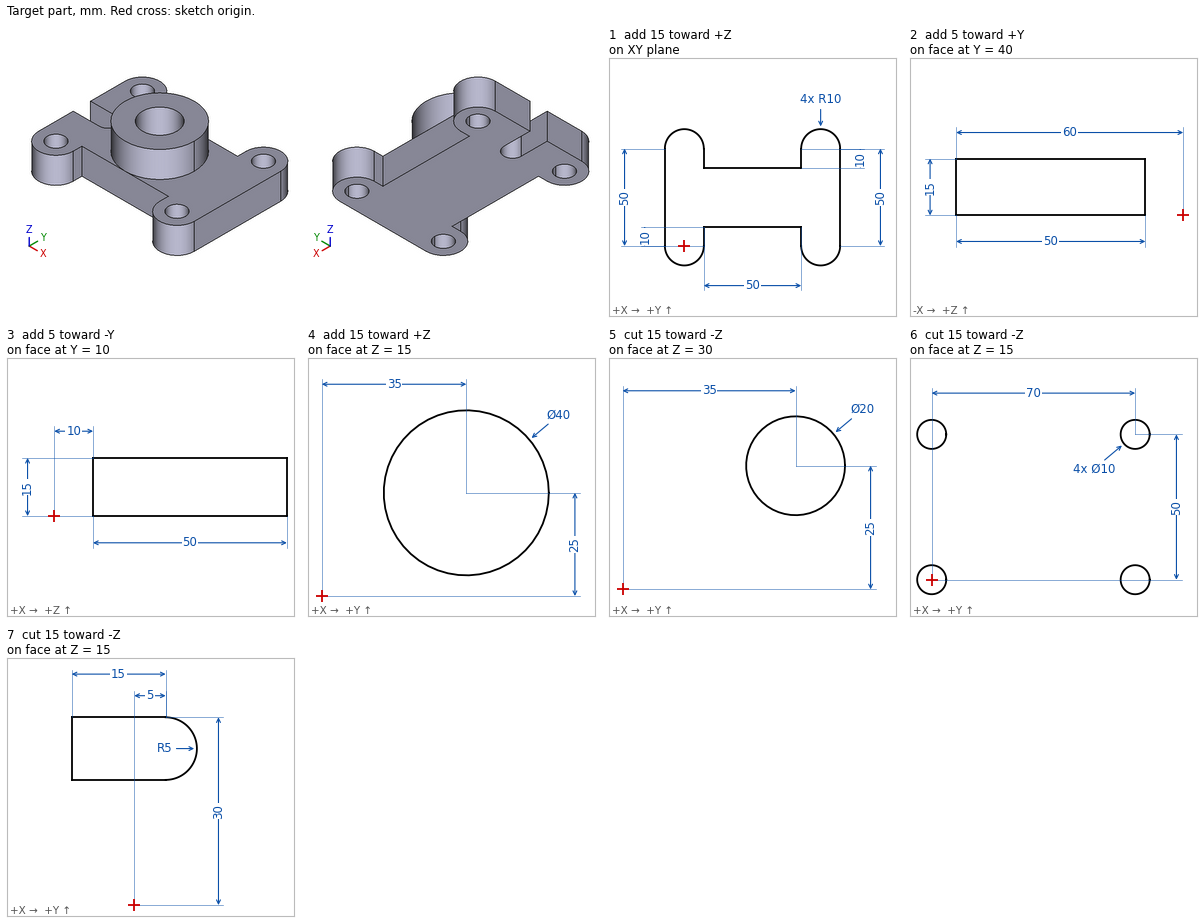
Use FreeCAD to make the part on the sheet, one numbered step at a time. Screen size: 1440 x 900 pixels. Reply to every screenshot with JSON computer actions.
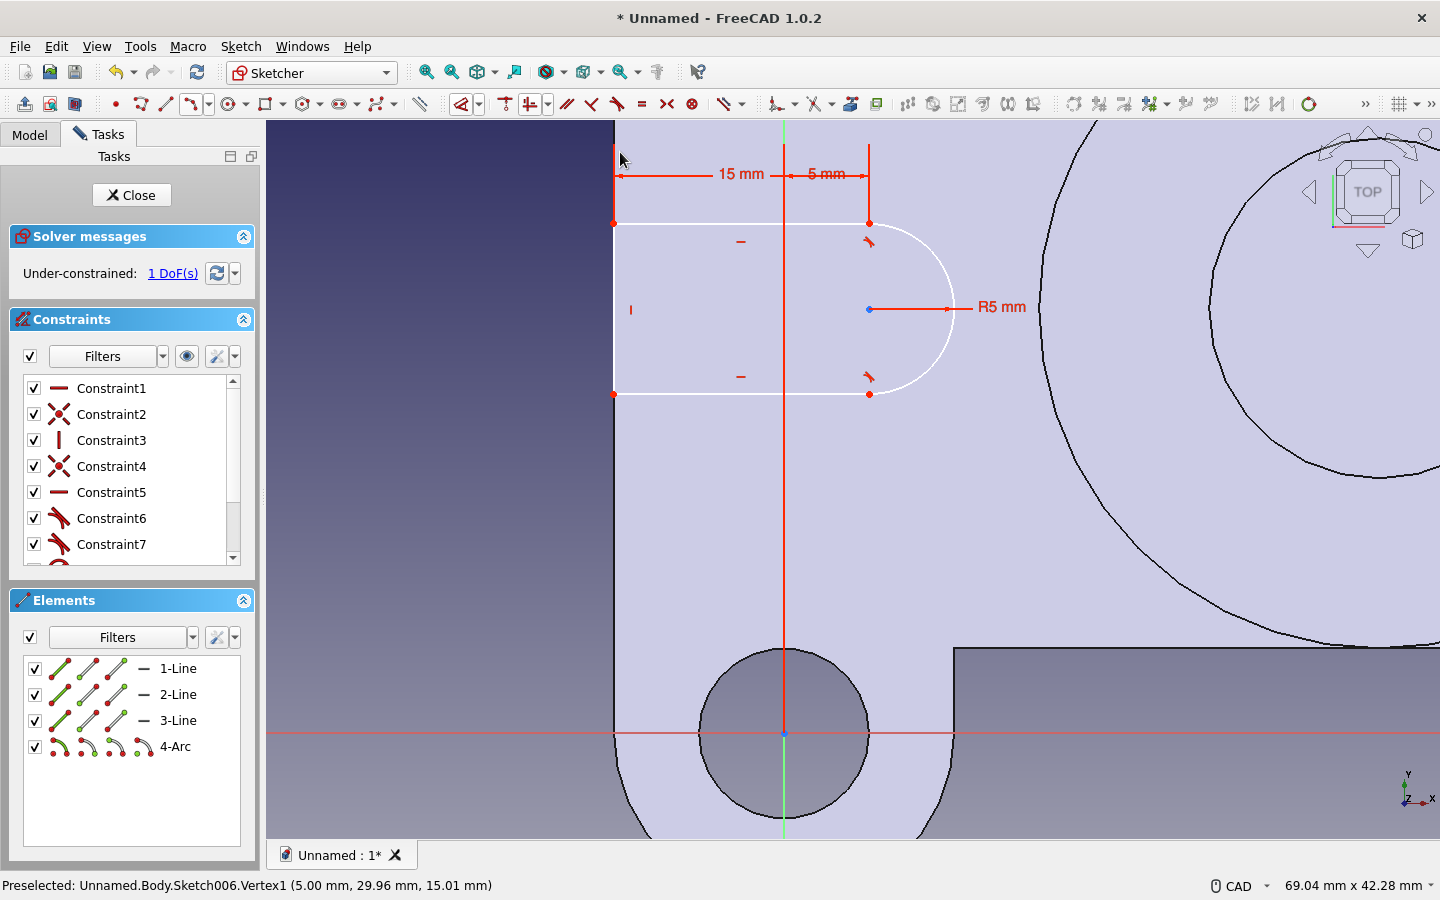
{"action": "left_click", "coordinate": [869, 224]}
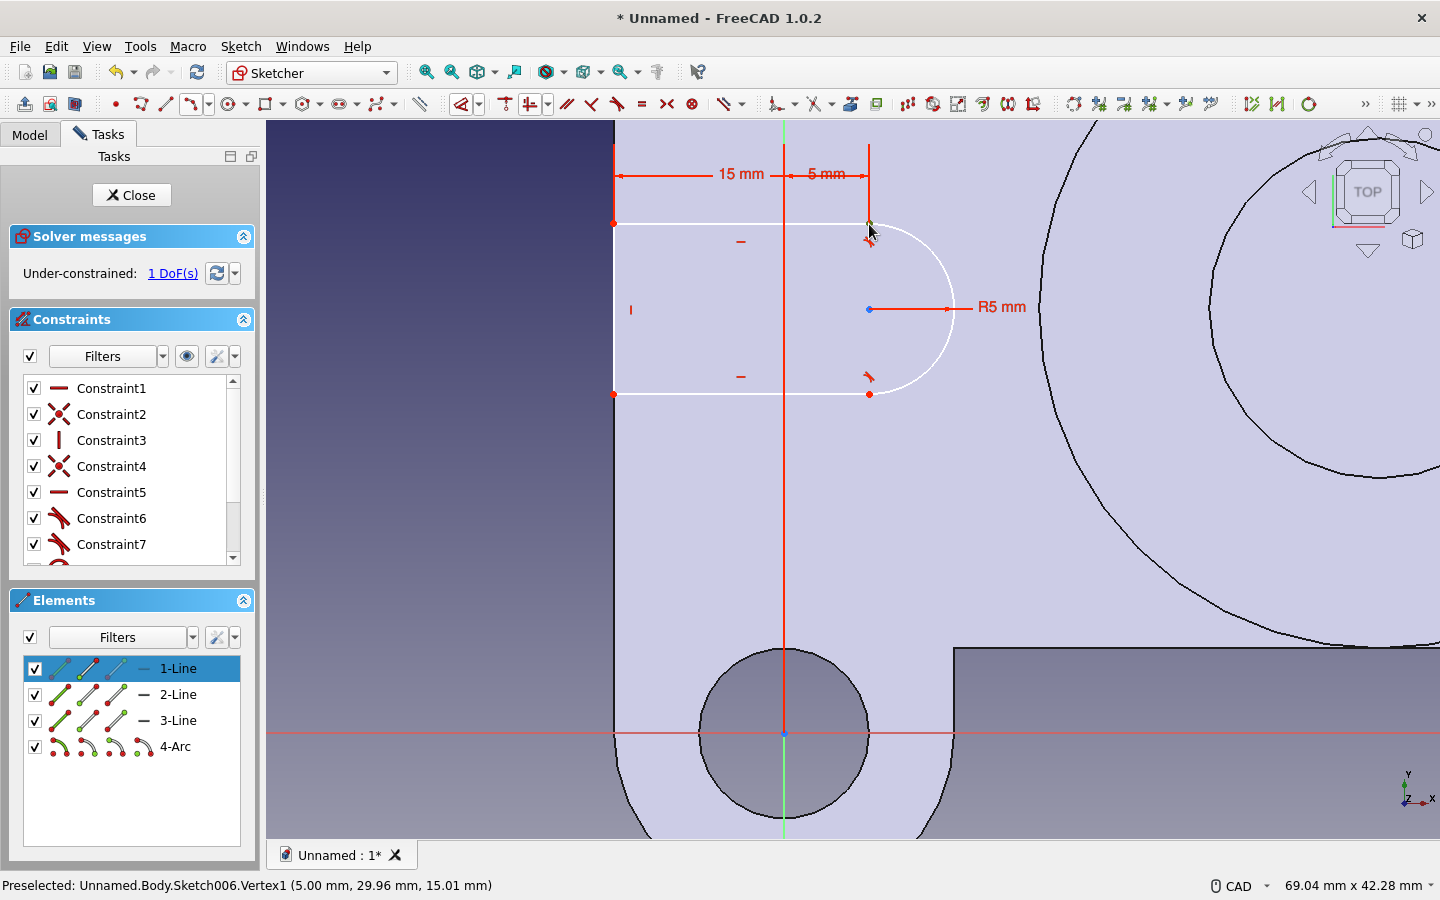
{"action": "key", "text": "i"}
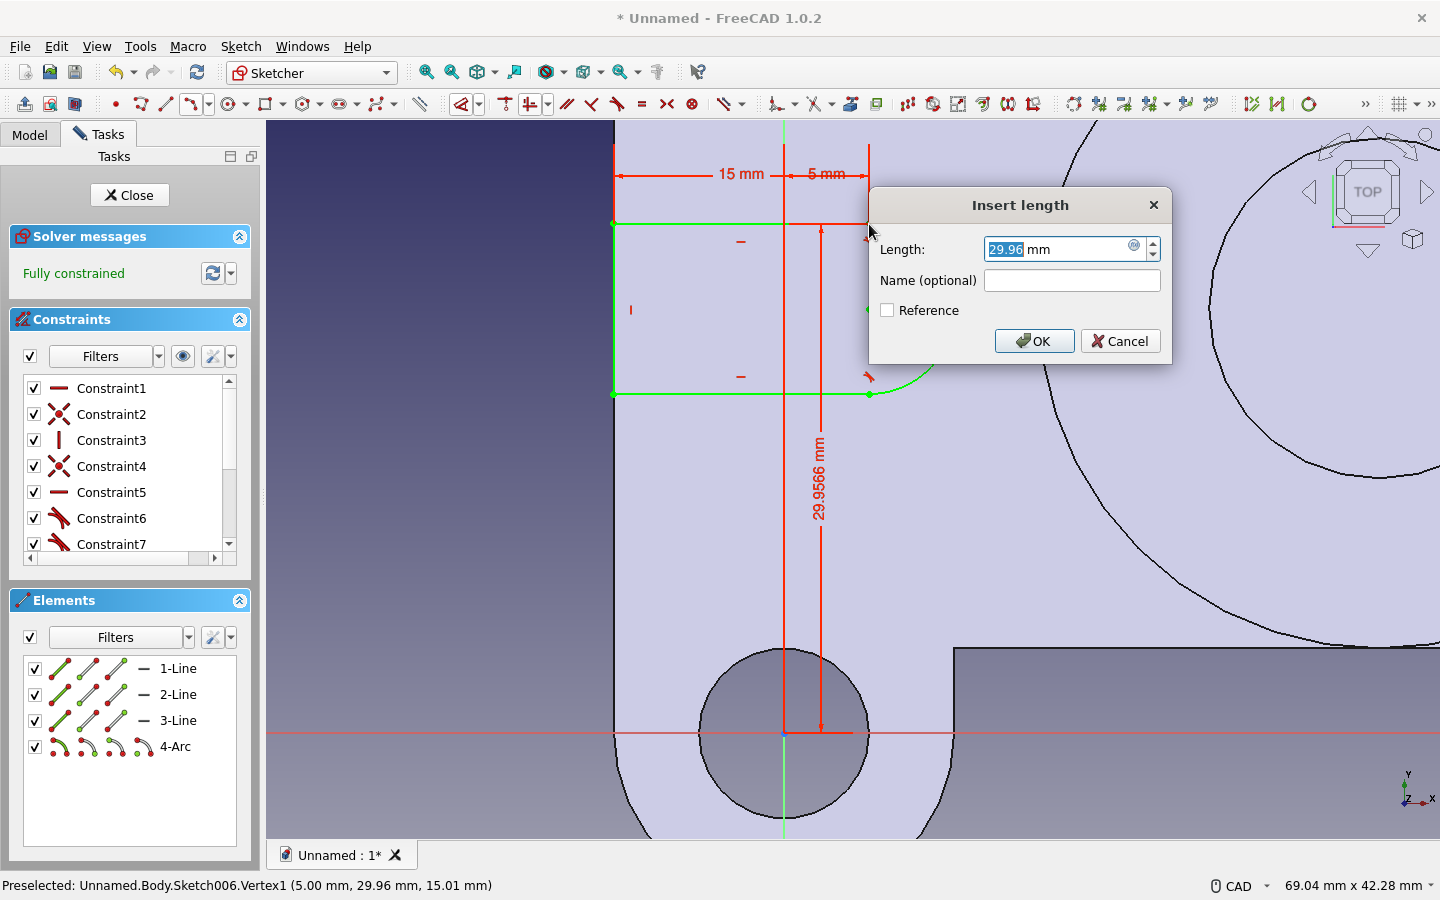
{"action": "type", "text": "30"}
{"action": "key", "text": "Return"}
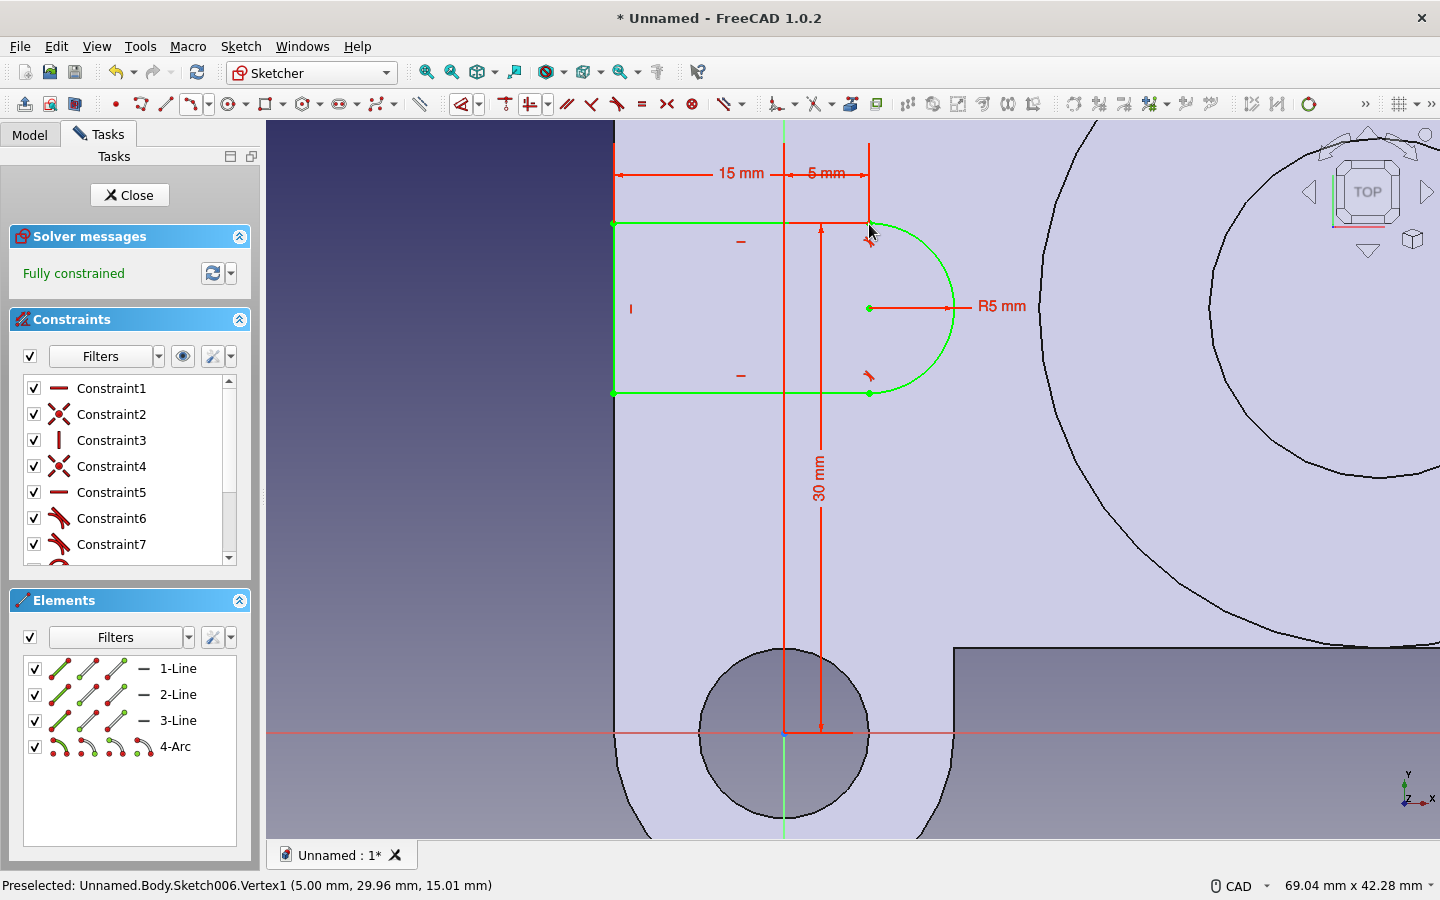
{"action": "left_click", "coordinate": [130, 195]}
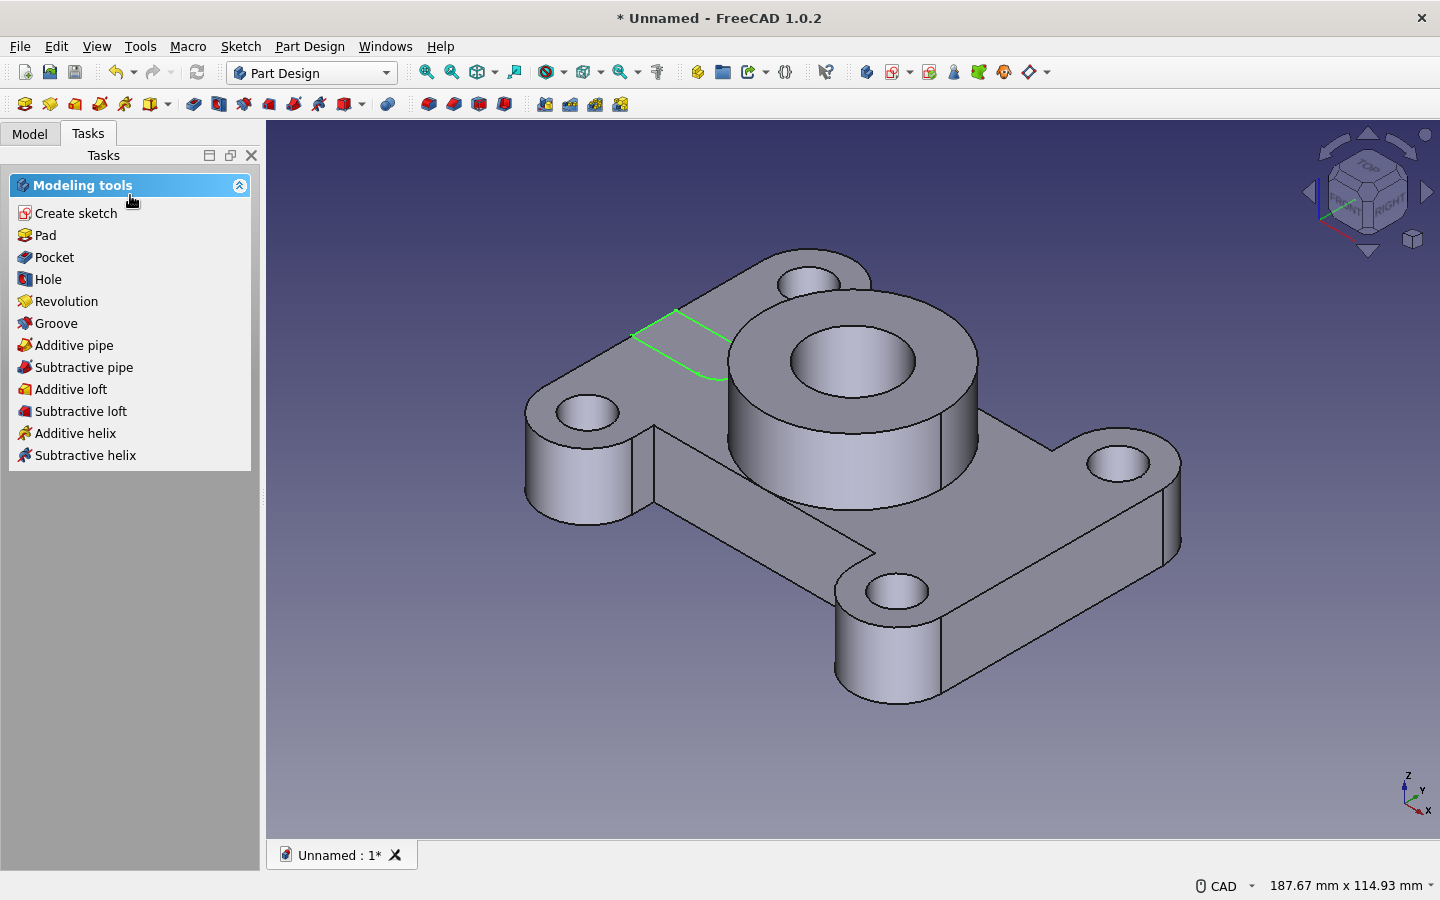
{"action": "left_click", "coordinate": [194, 104]}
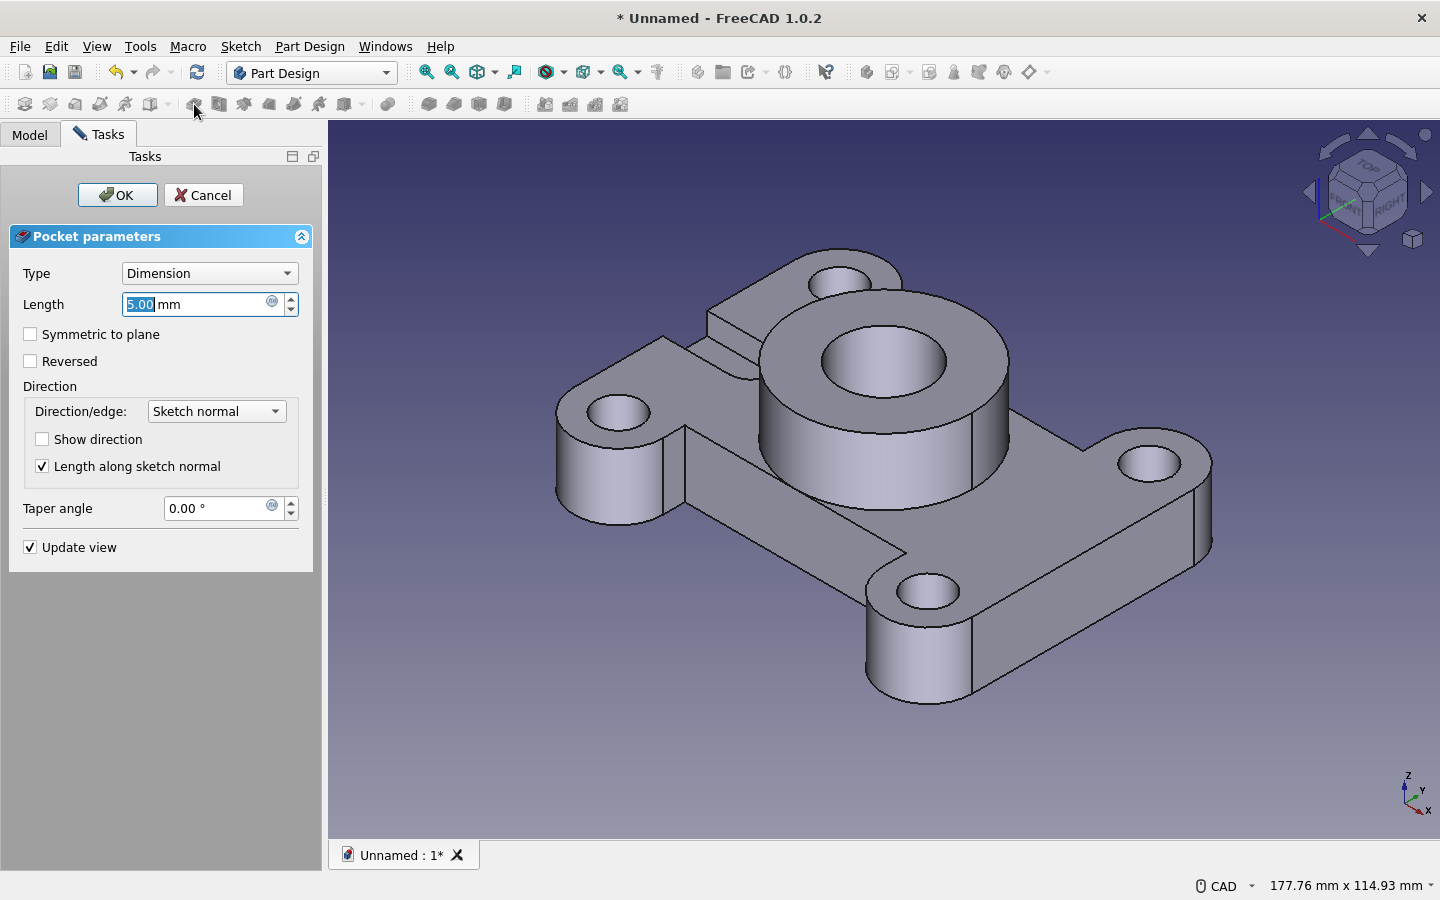
{"action": "type", "text": "15"}
{"action": "key", "text": "Tab"}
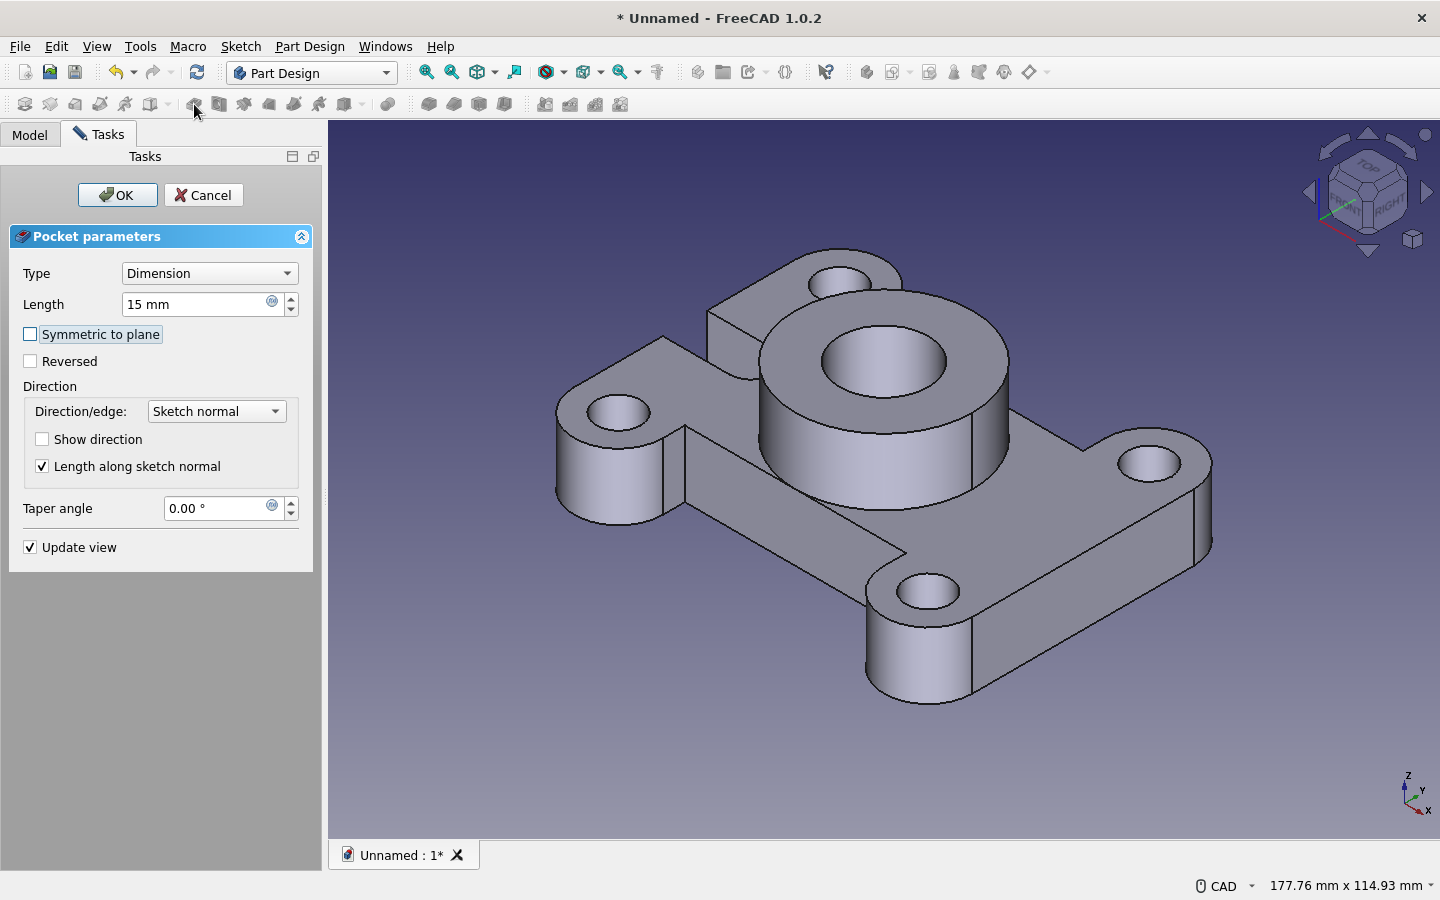
{"action": "left_click", "coordinate": [118, 195]}